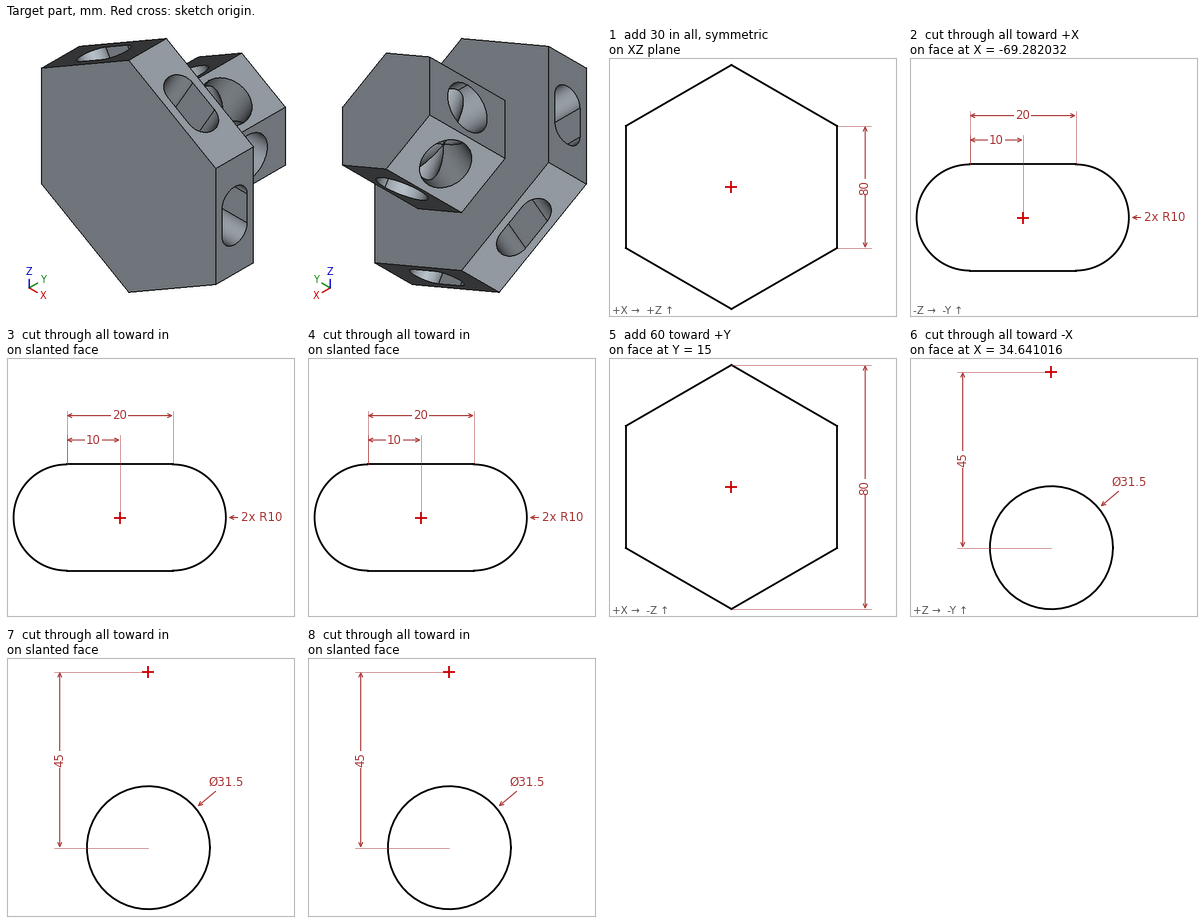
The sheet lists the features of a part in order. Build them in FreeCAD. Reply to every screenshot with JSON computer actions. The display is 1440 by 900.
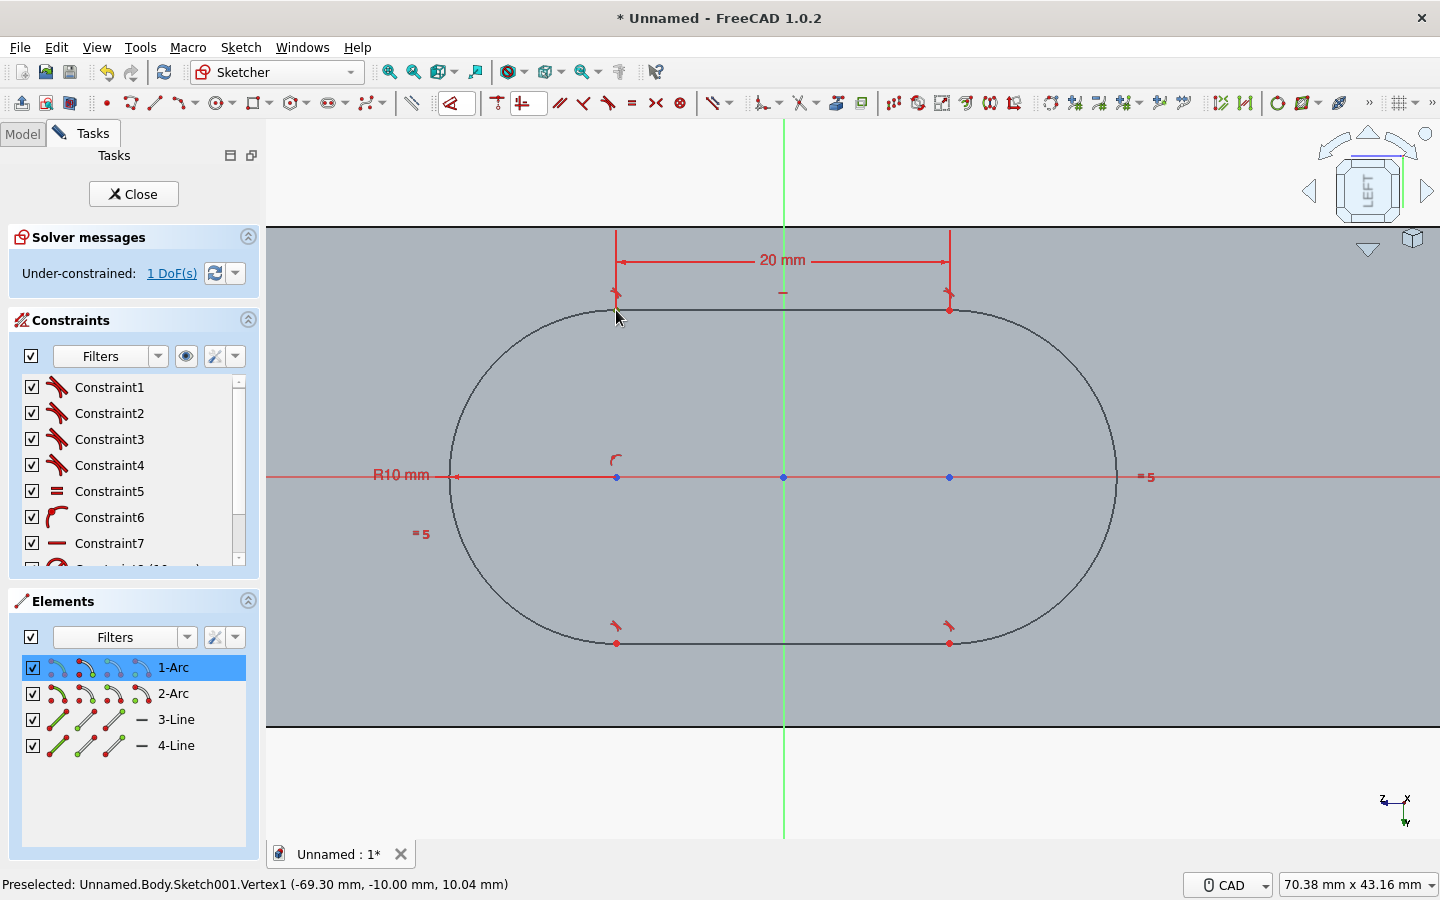
{"action": "key", "text": "l"}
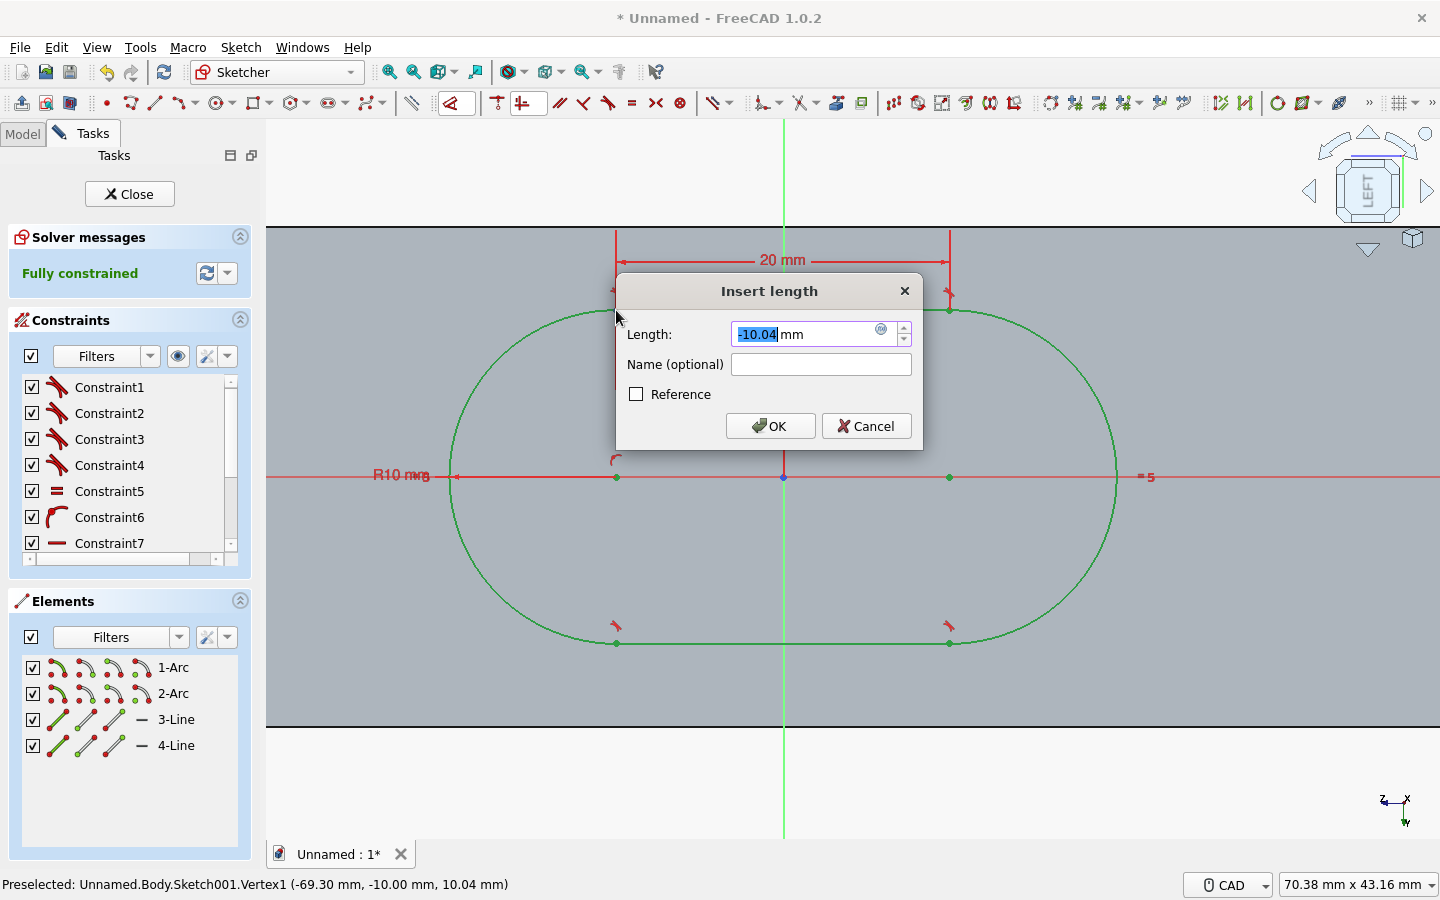
{"action": "type", "text": "-10"}
{"action": "key", "text": "Return"}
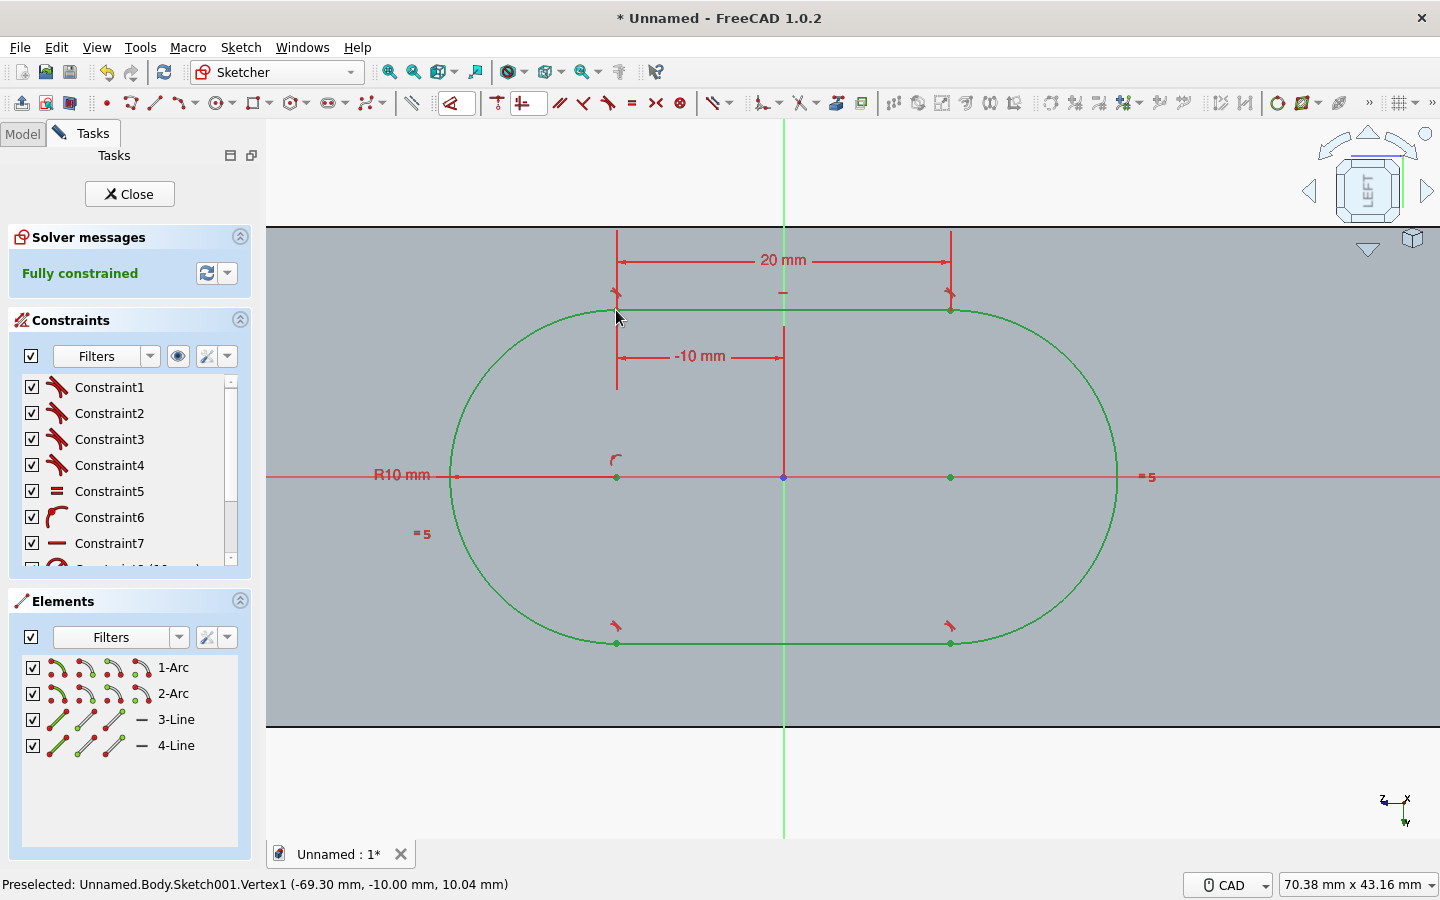
{"action": "left_click", "coordinate": [130, 194]}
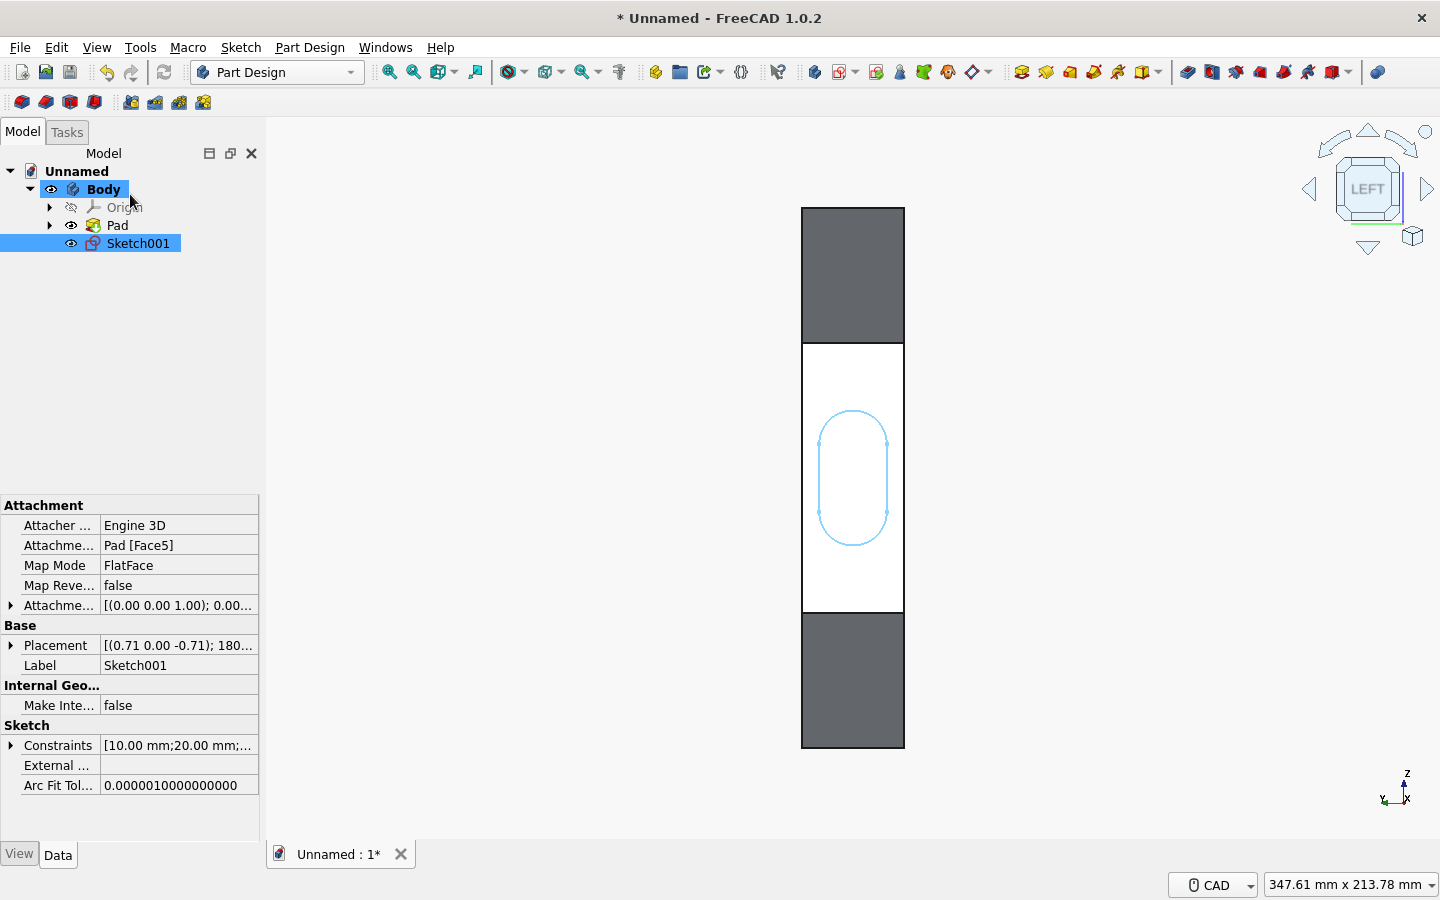
{"action": "left_click", "coordinate": [1188, 72]}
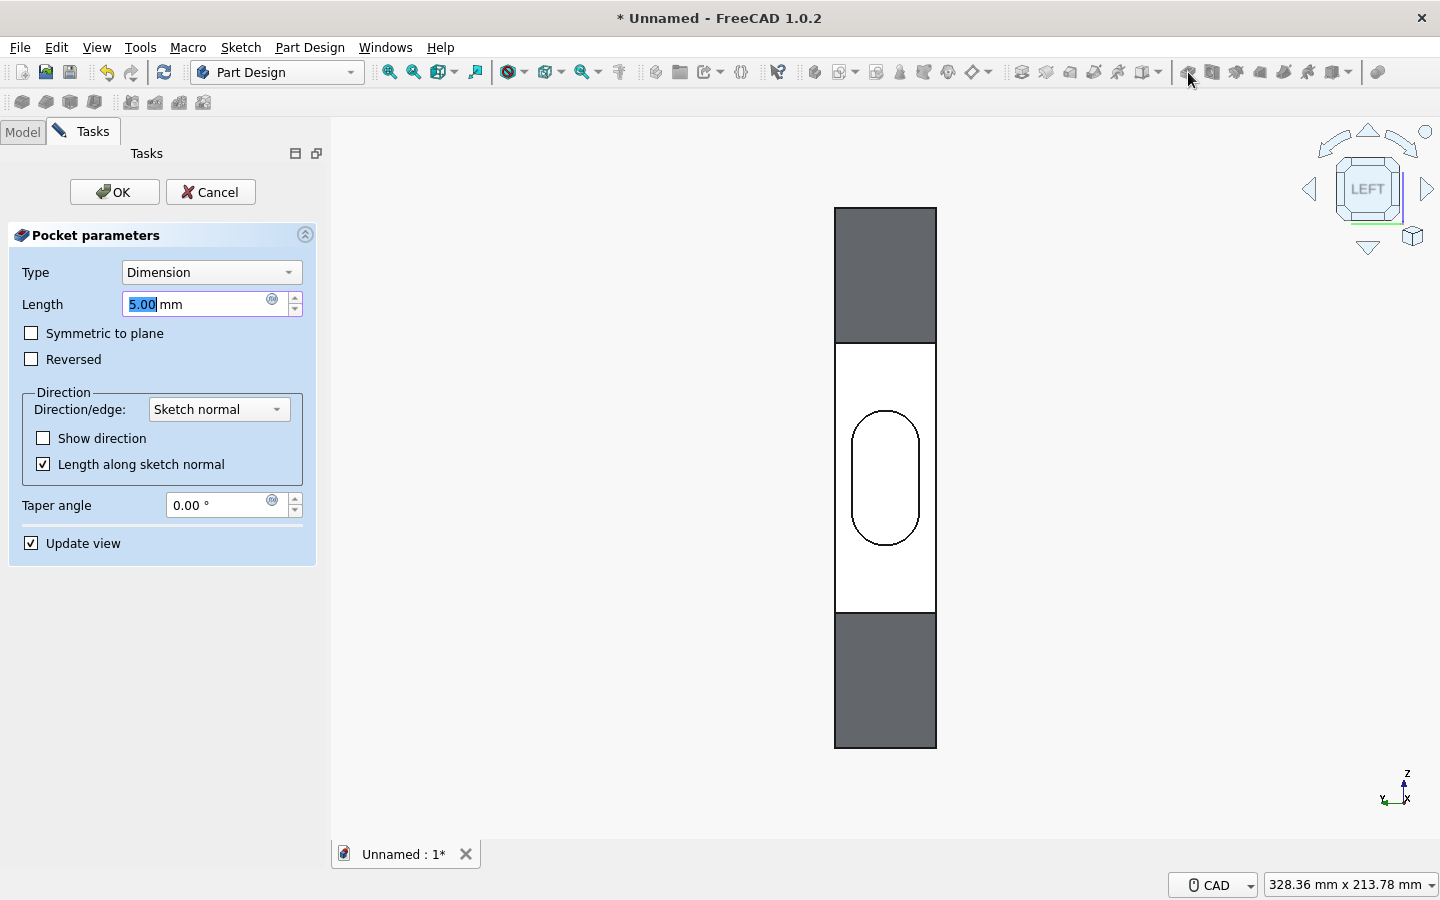
{"action": "left_click", "coordinate": [212, 272]}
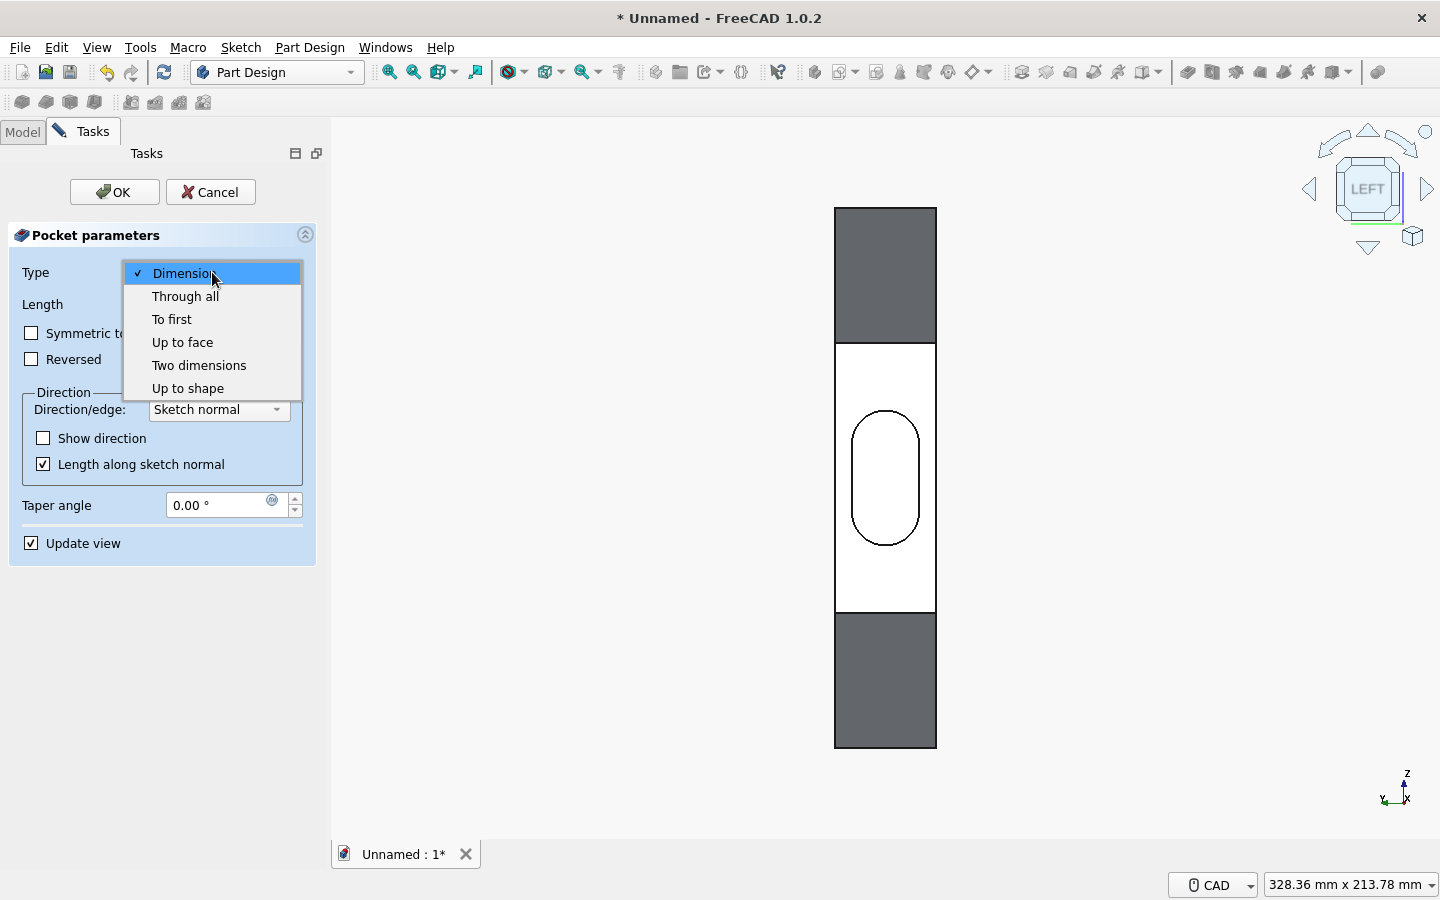
{"action": "left_click", "coordinate": [212, 296]}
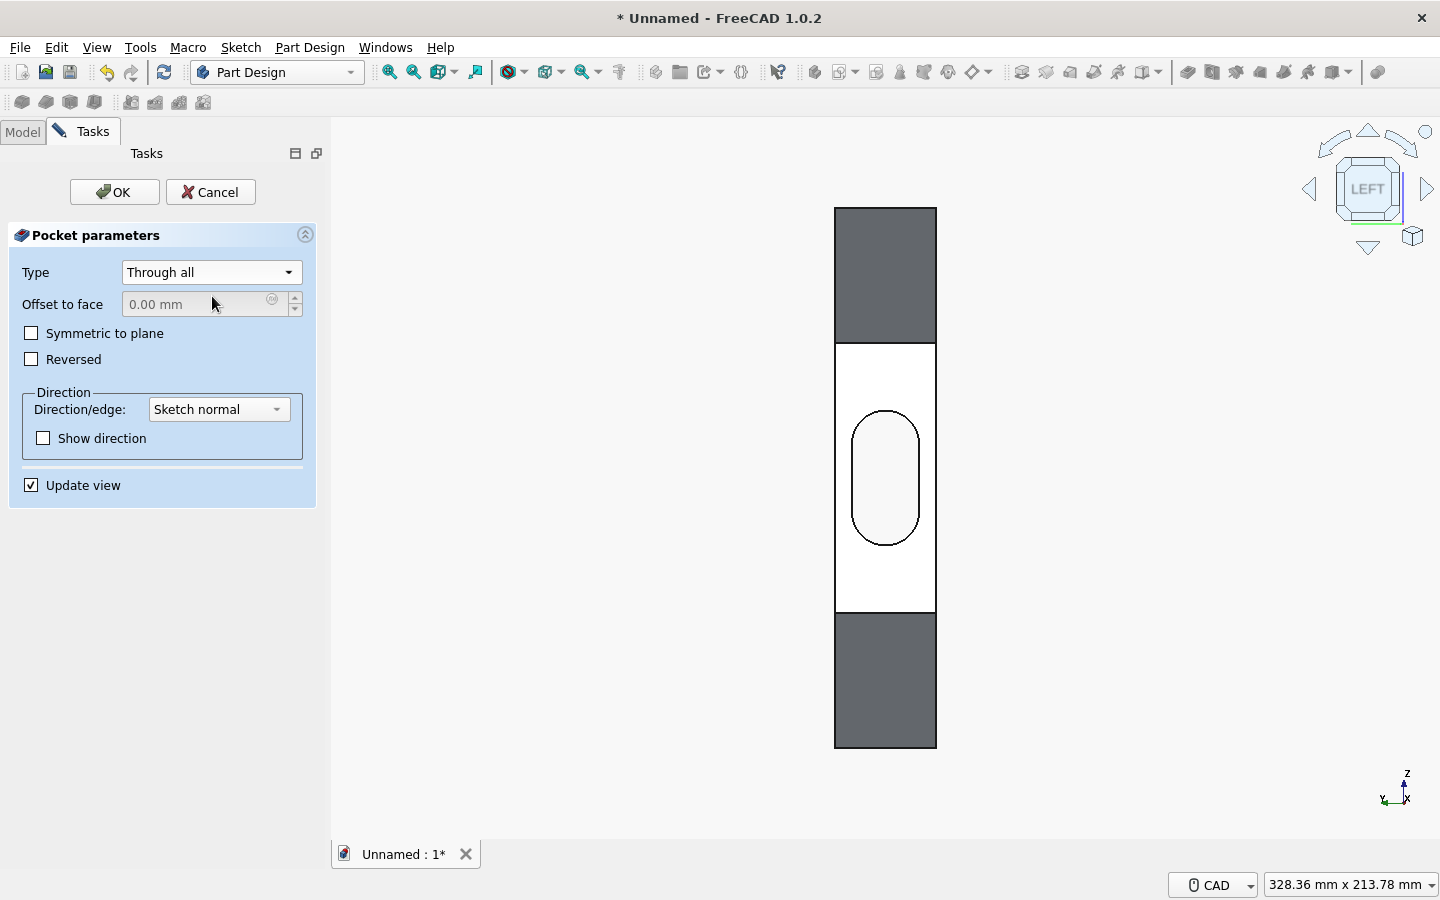
{"action": "left_click", "coordinate": [115, 192]}